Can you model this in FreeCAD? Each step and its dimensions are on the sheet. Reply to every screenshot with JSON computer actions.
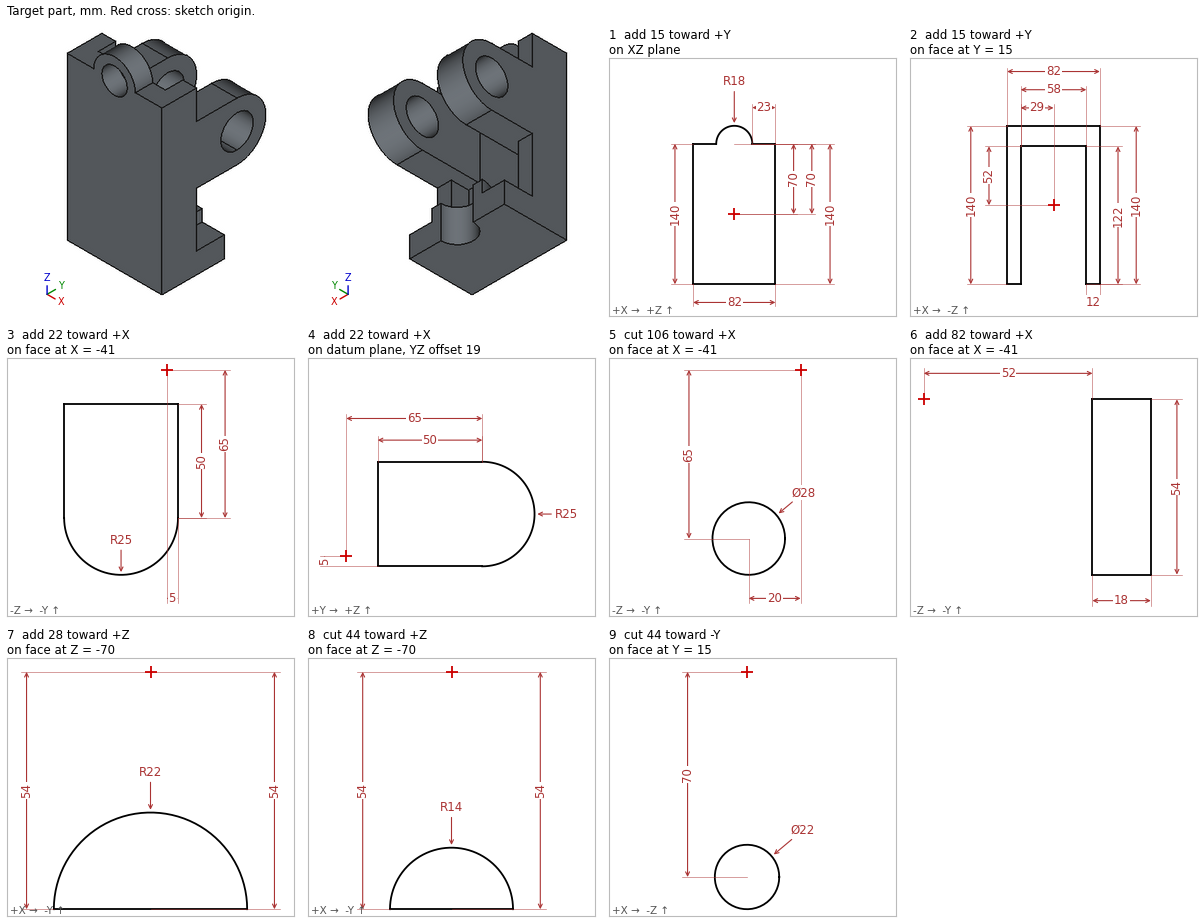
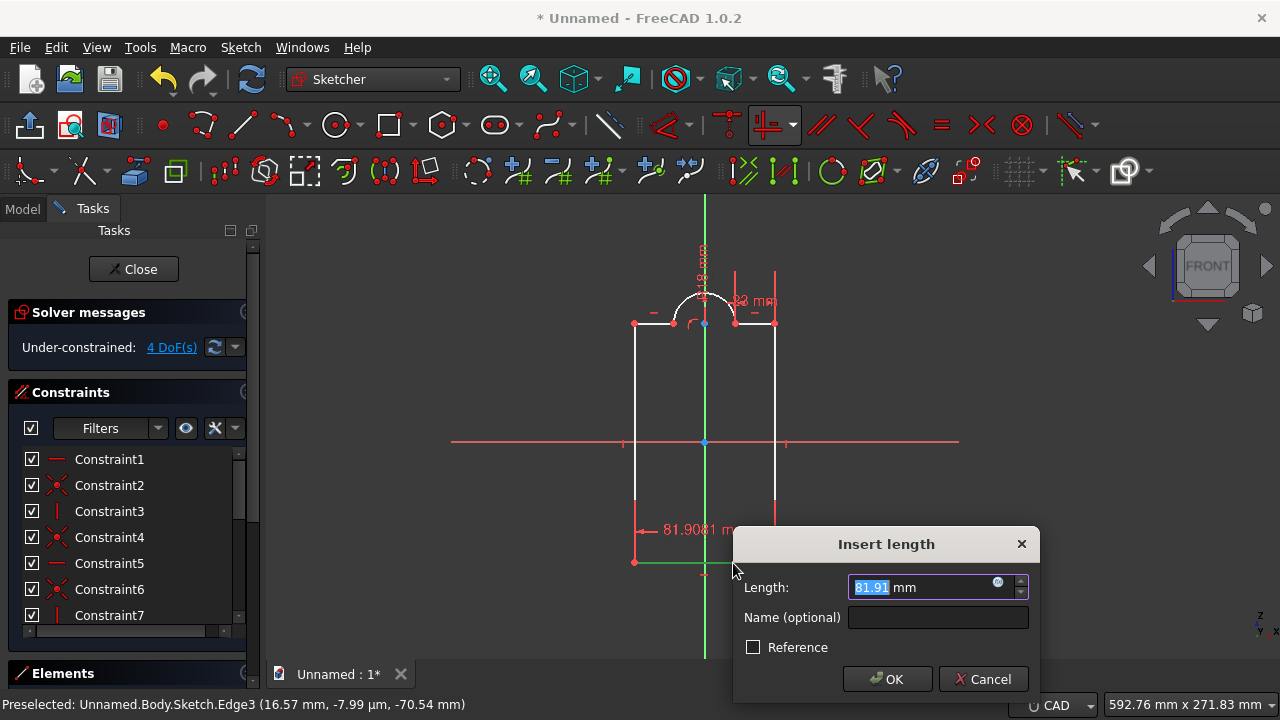
{"action": "type", "text": "82"}
{"action": "key", "text": "Return"}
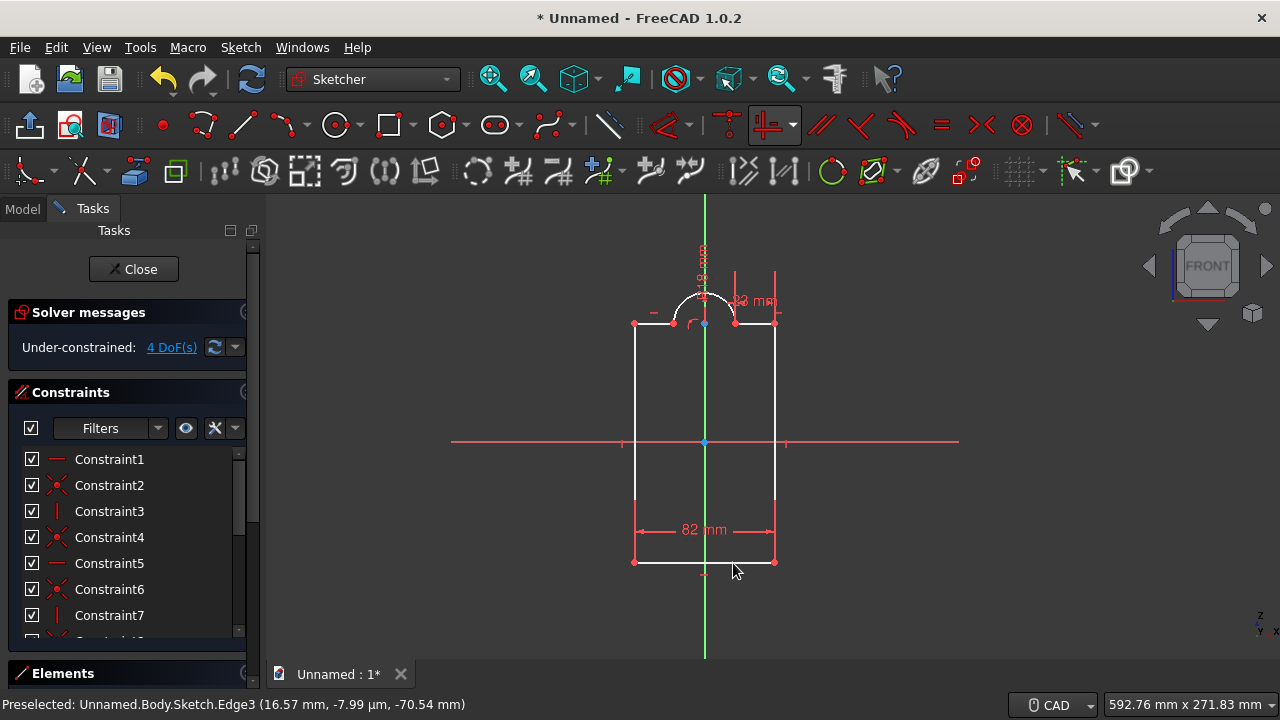
{"action": "left_click", "coordinate": [775, 395]}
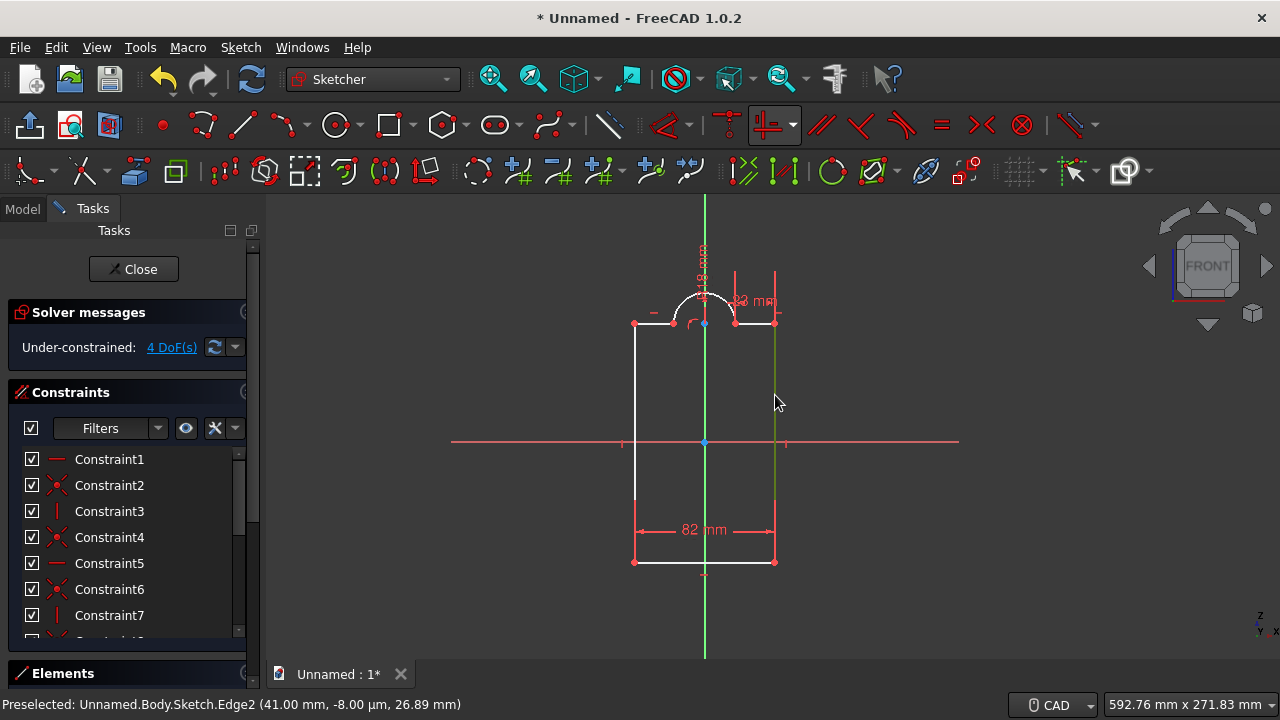
{"action": "key", "text": "i"}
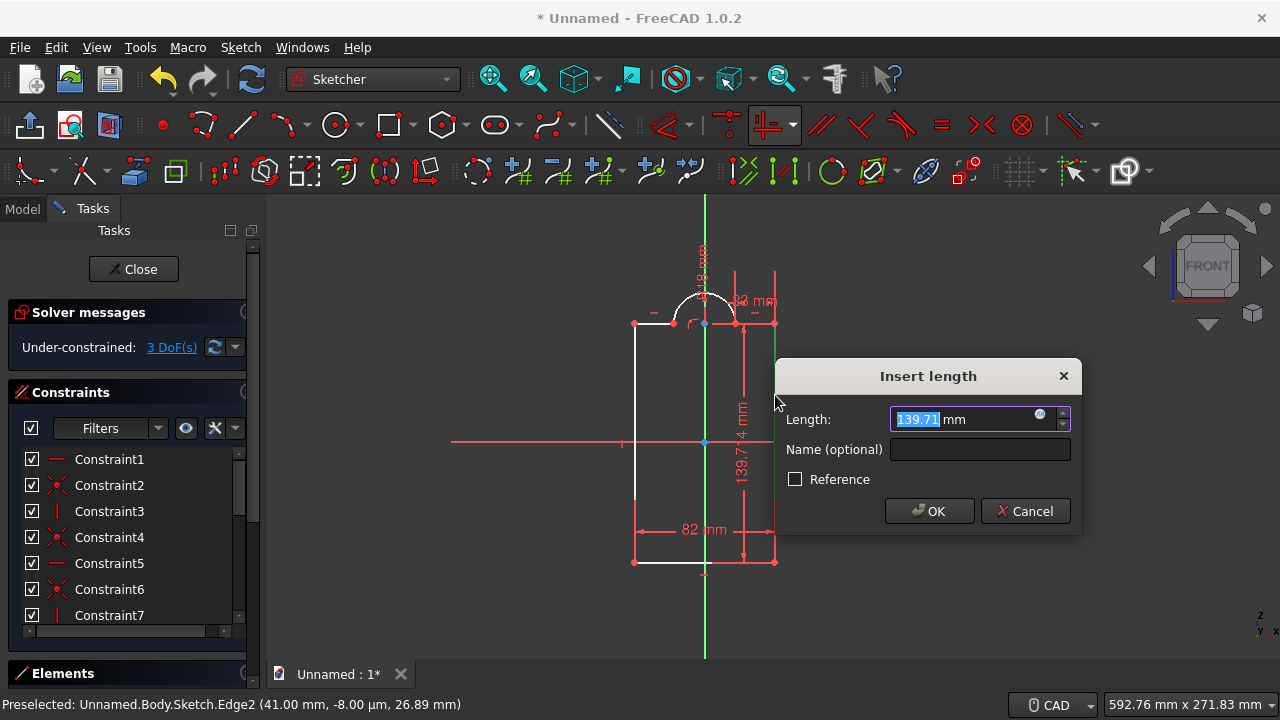
{"action": "type", "text": "140"}
{"action": "key", "text": "Return"}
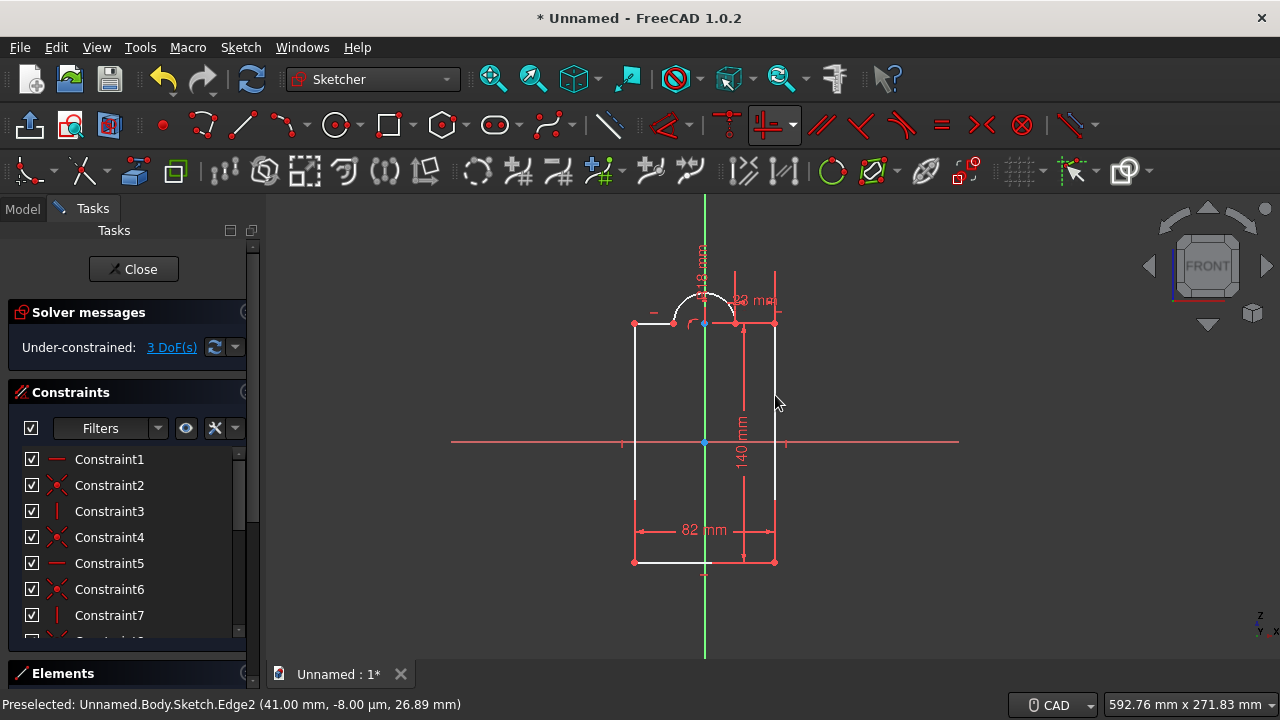
{"action": "left_click", "coordinate": [635, 491]}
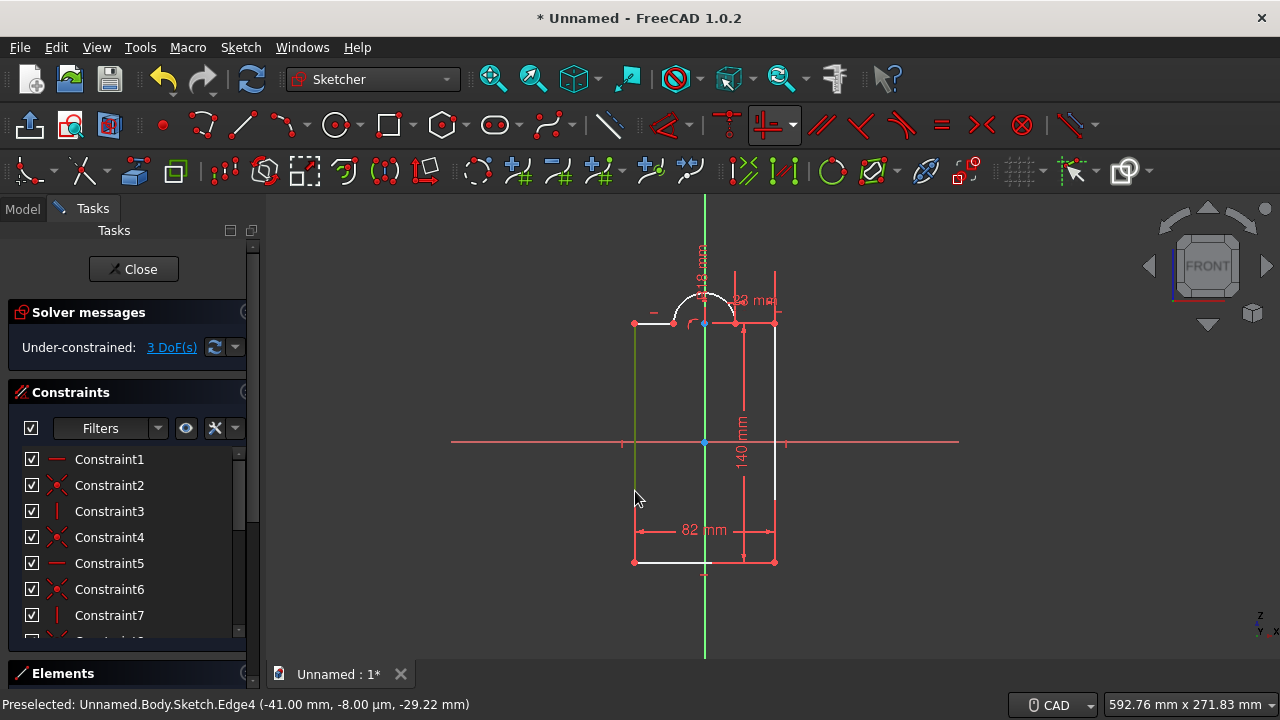
{"action": "key", "text": "i"}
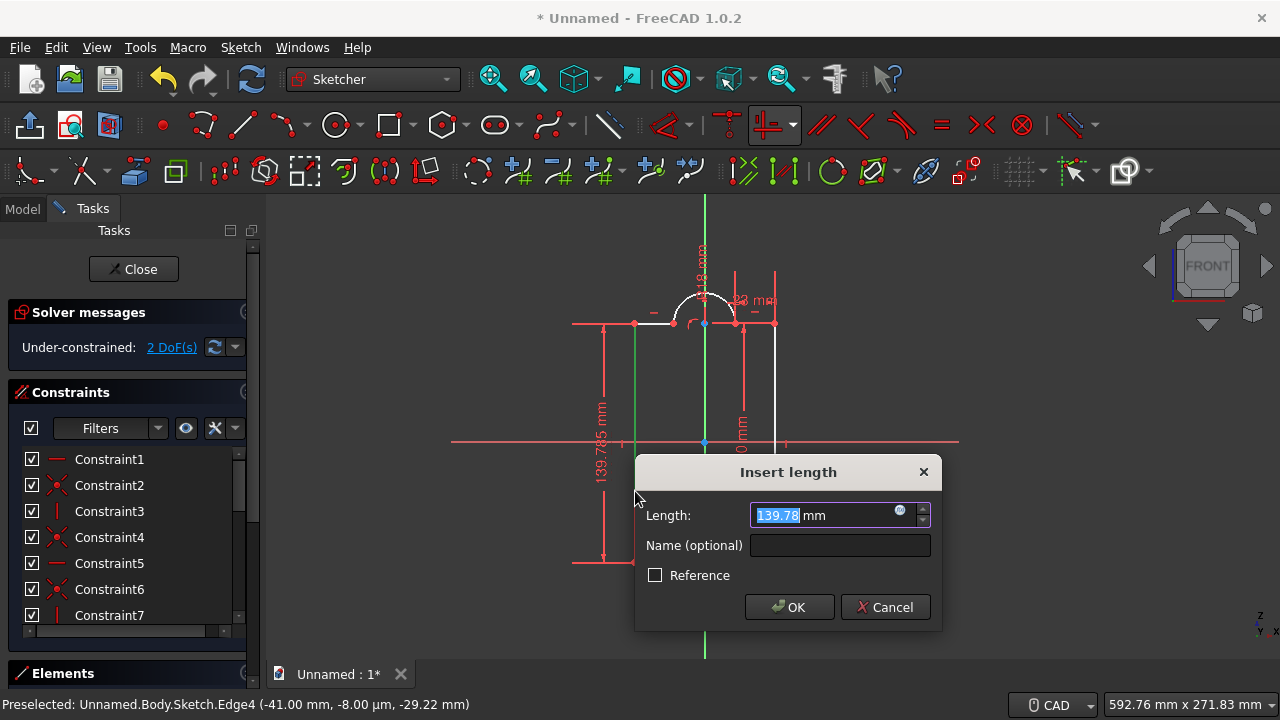
{"action": "type", "text": "140"}
{"action": "key", "text": "Return"}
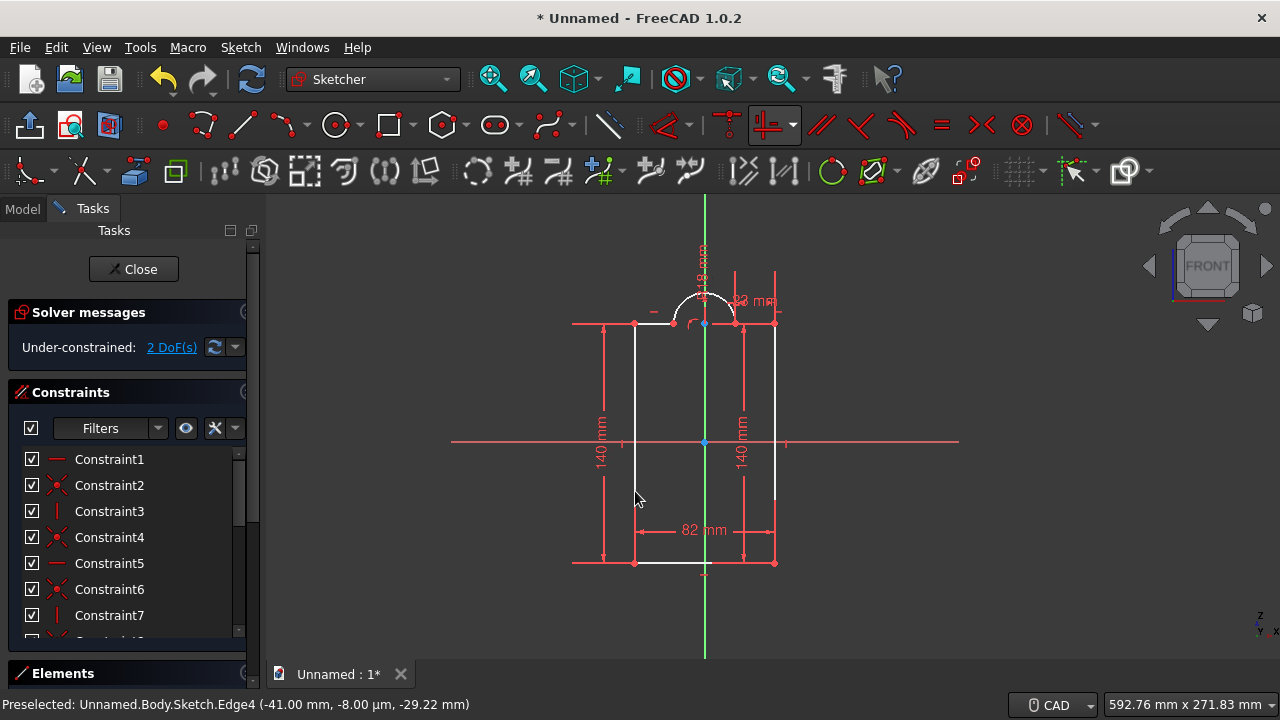
{"action": "left_click", "coordinate": [735, 324]}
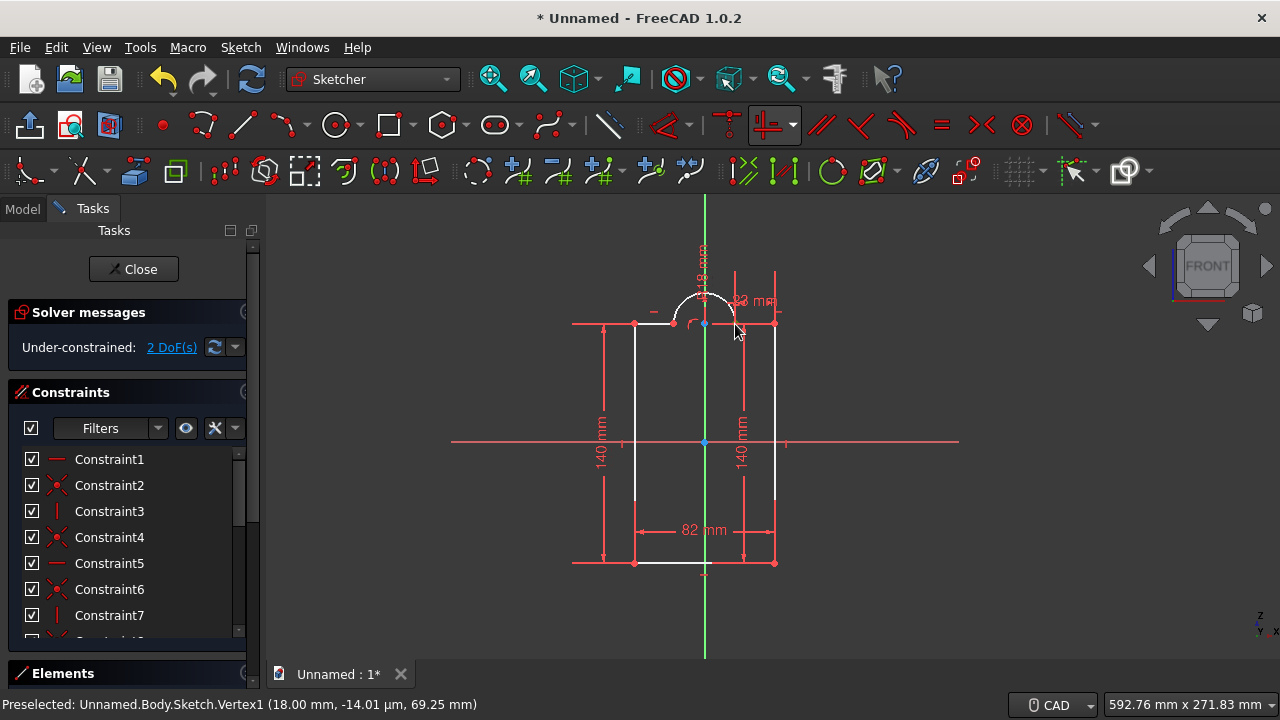
{"action": "key", "text": "i"}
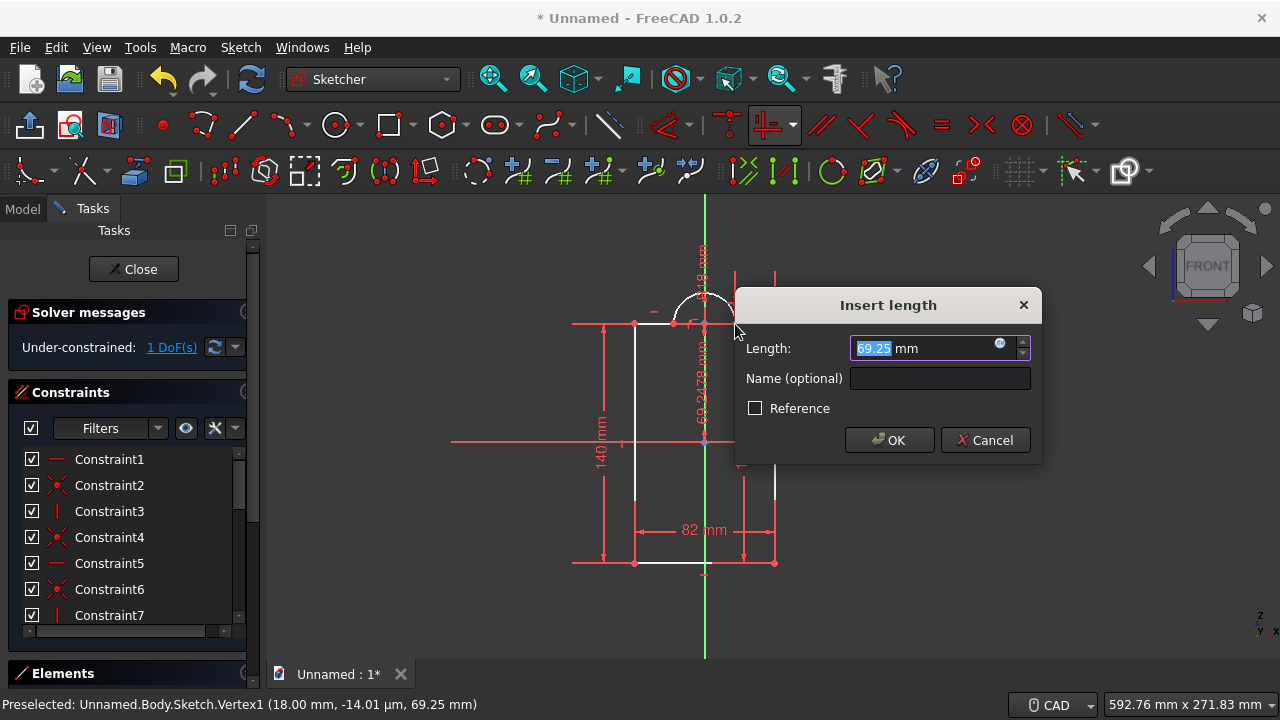
{"action": "type", "text": "70"}
{"action": "key", "text": "Return"}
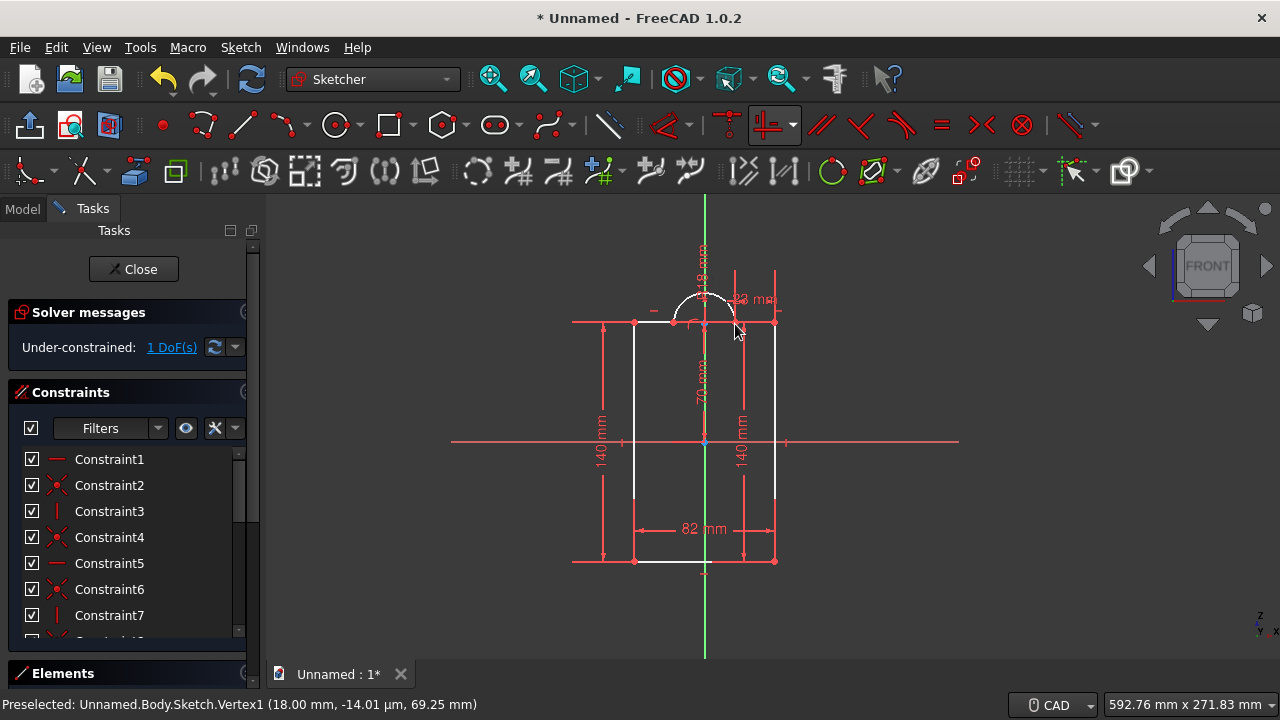
{"action": "left_click", "coordinate": [705, 324]}